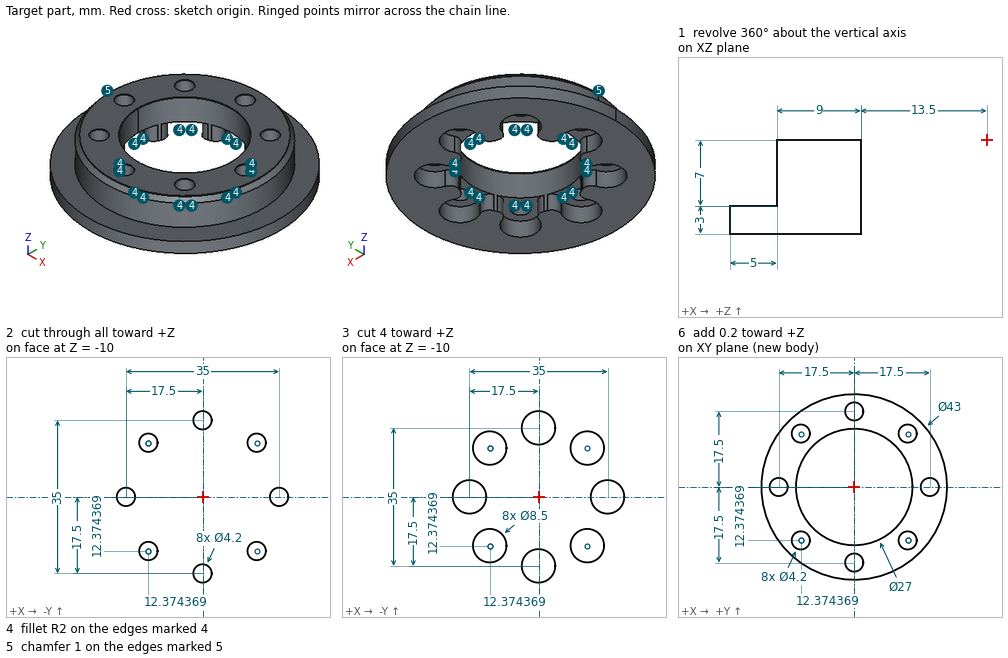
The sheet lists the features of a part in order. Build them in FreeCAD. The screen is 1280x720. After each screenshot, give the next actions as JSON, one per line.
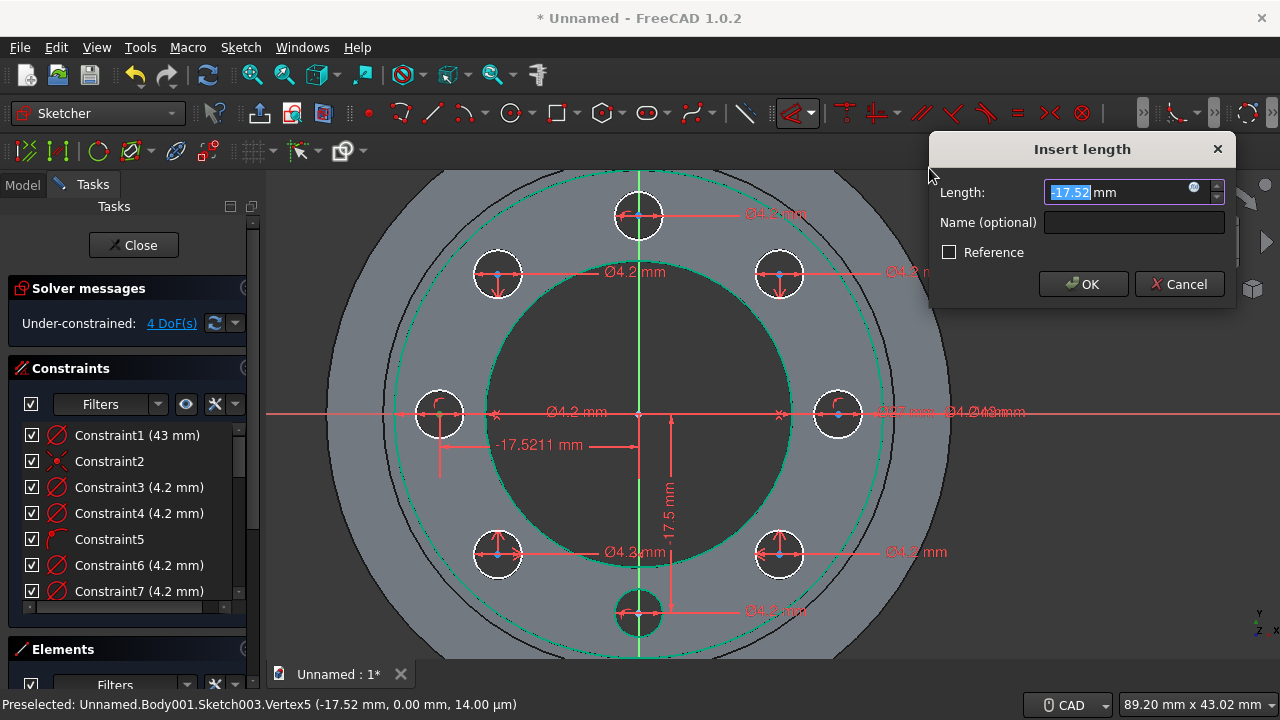
{"action": "type", "text": "-17.5"}
{"action": "key", "text": "Return"}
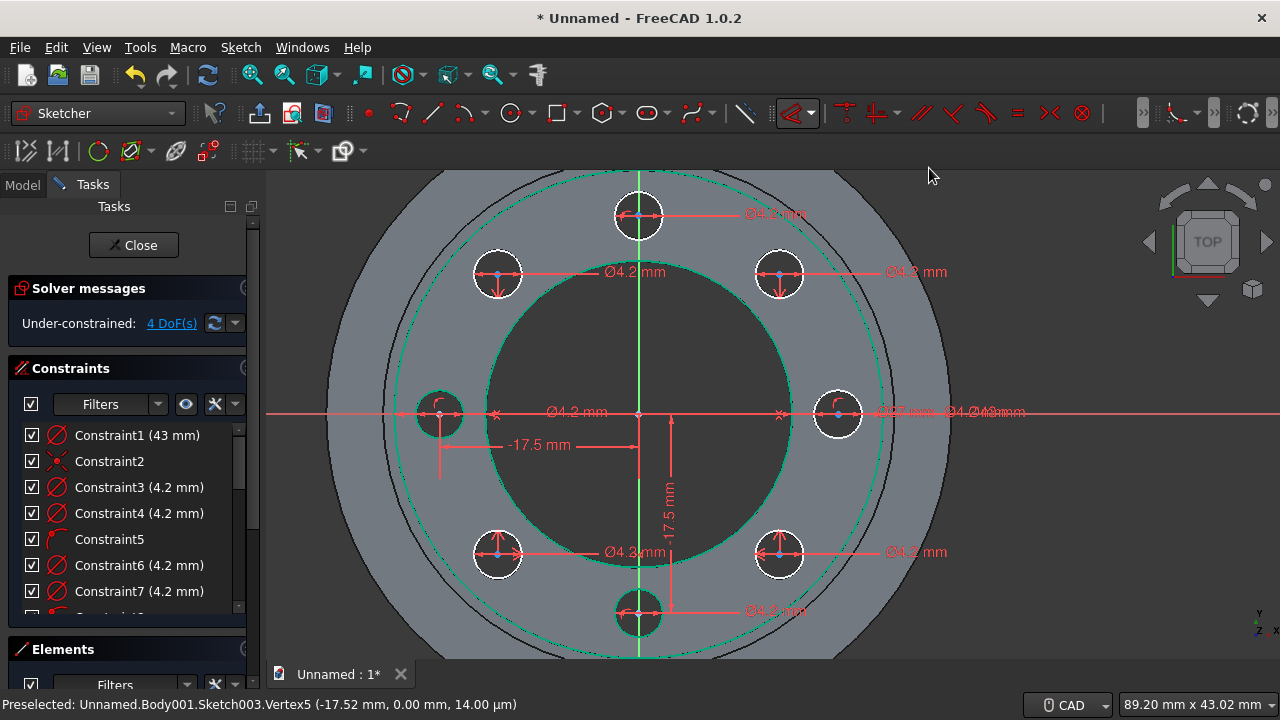
{"action": "left_click", "coordinate": [838, 414]}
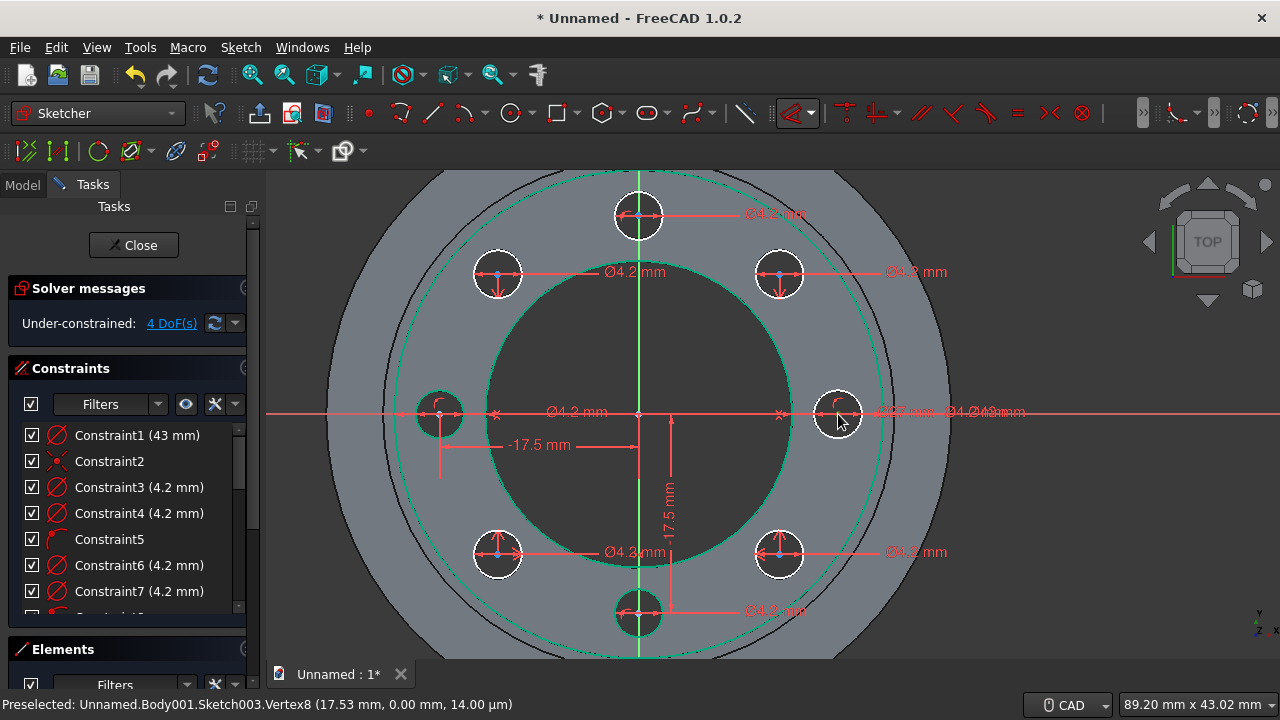
{"action": "key", "text": "l"}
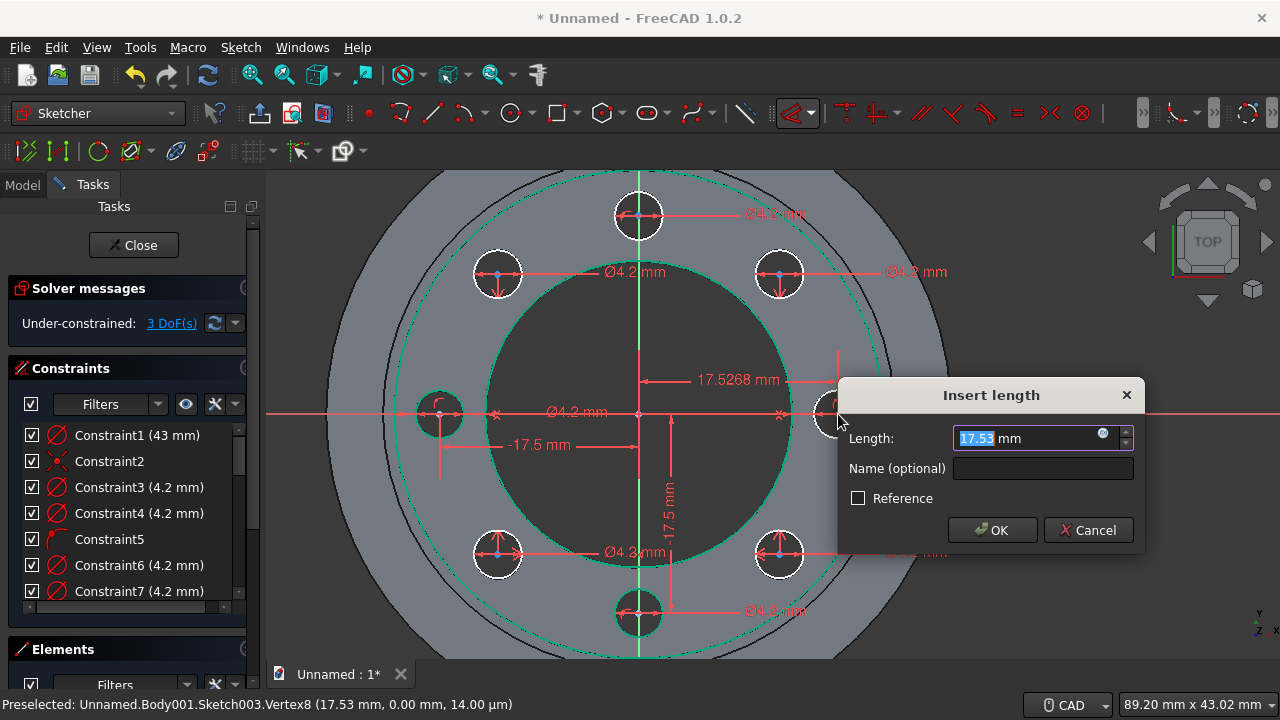
{"action": "type", "text": "17.5"}
{"action": "key", "text": "Return"}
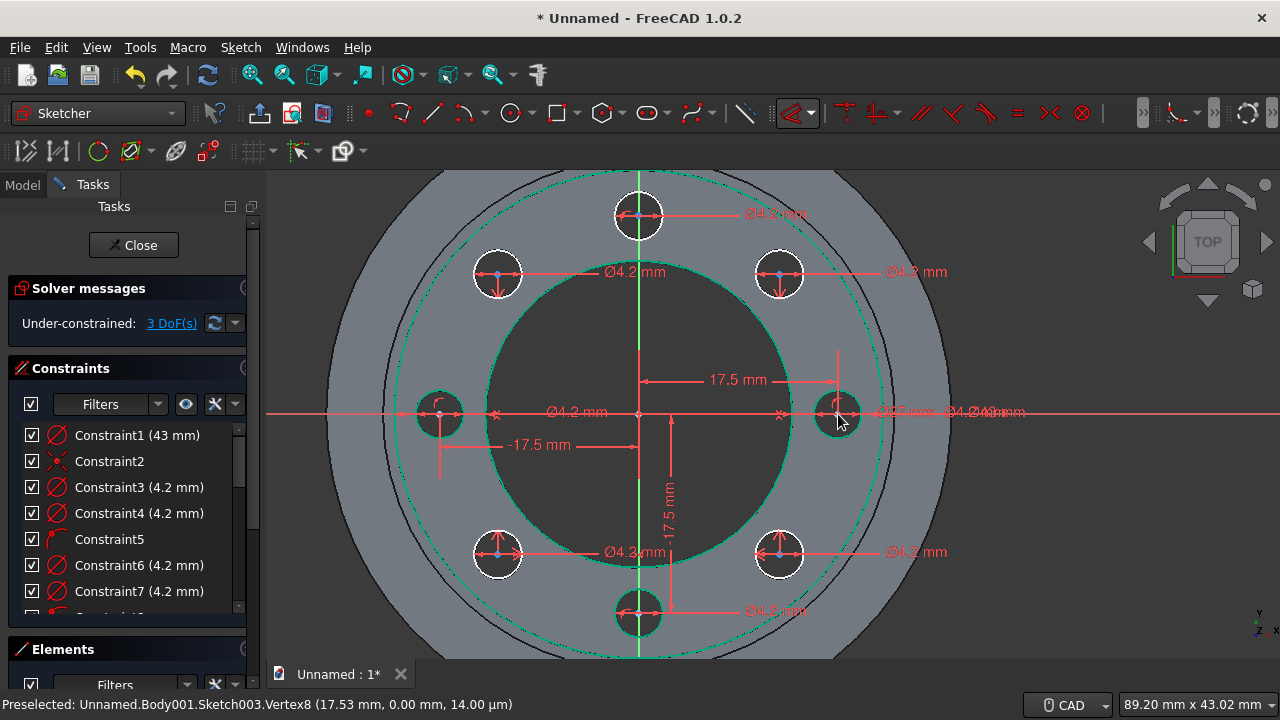
{"action": "left_click", "coordinate": [639, 216]}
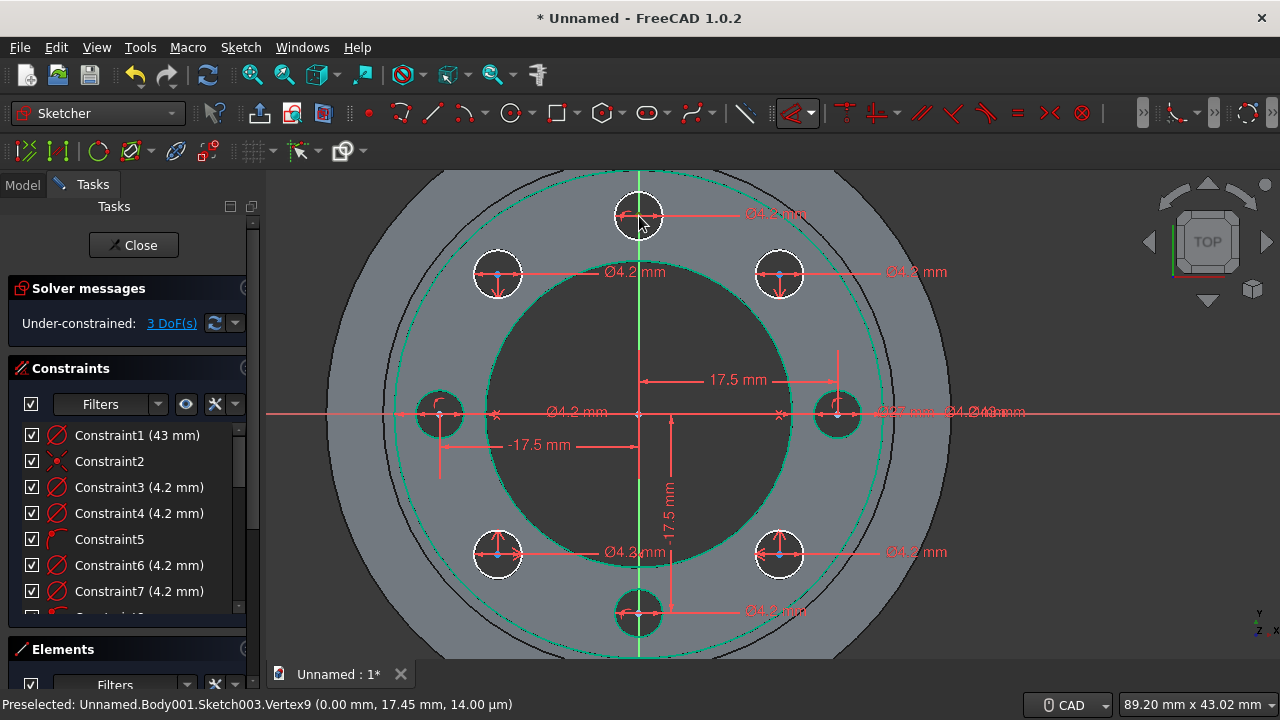
{"action": "key", "text": "i"}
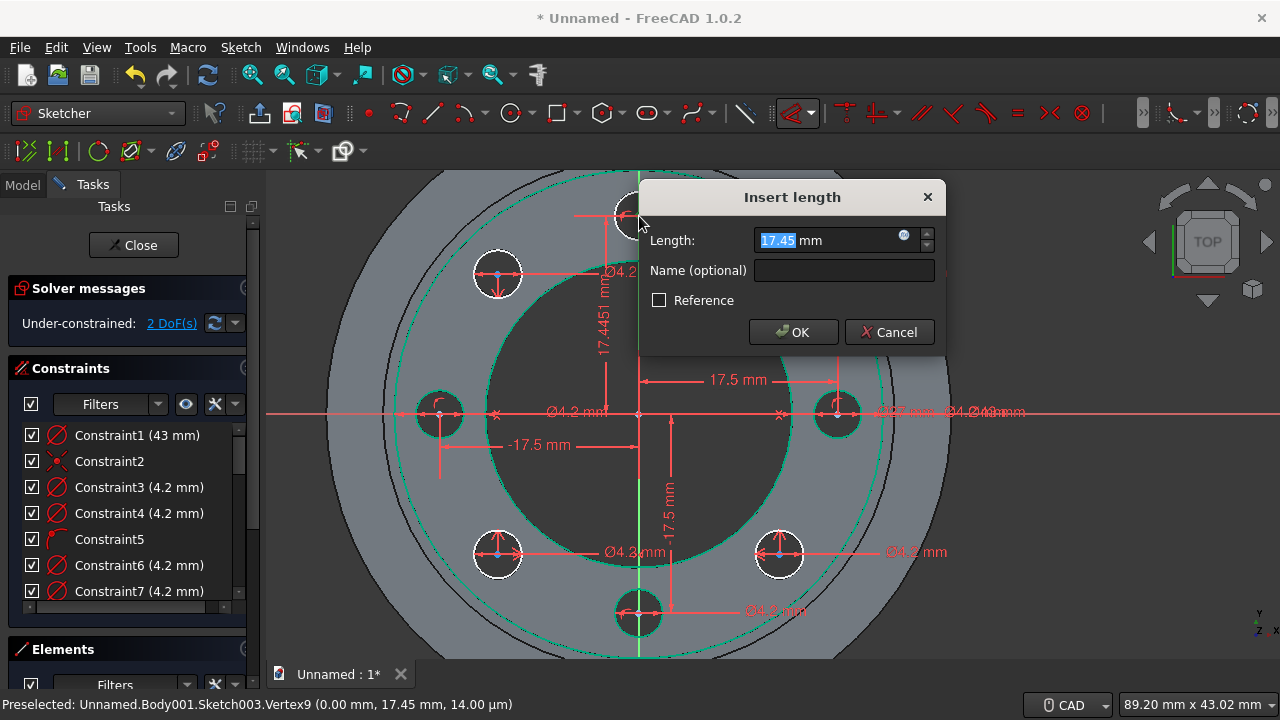
{"action": "type", "text": "17.5"}
{"action": "key", "text": "Return"}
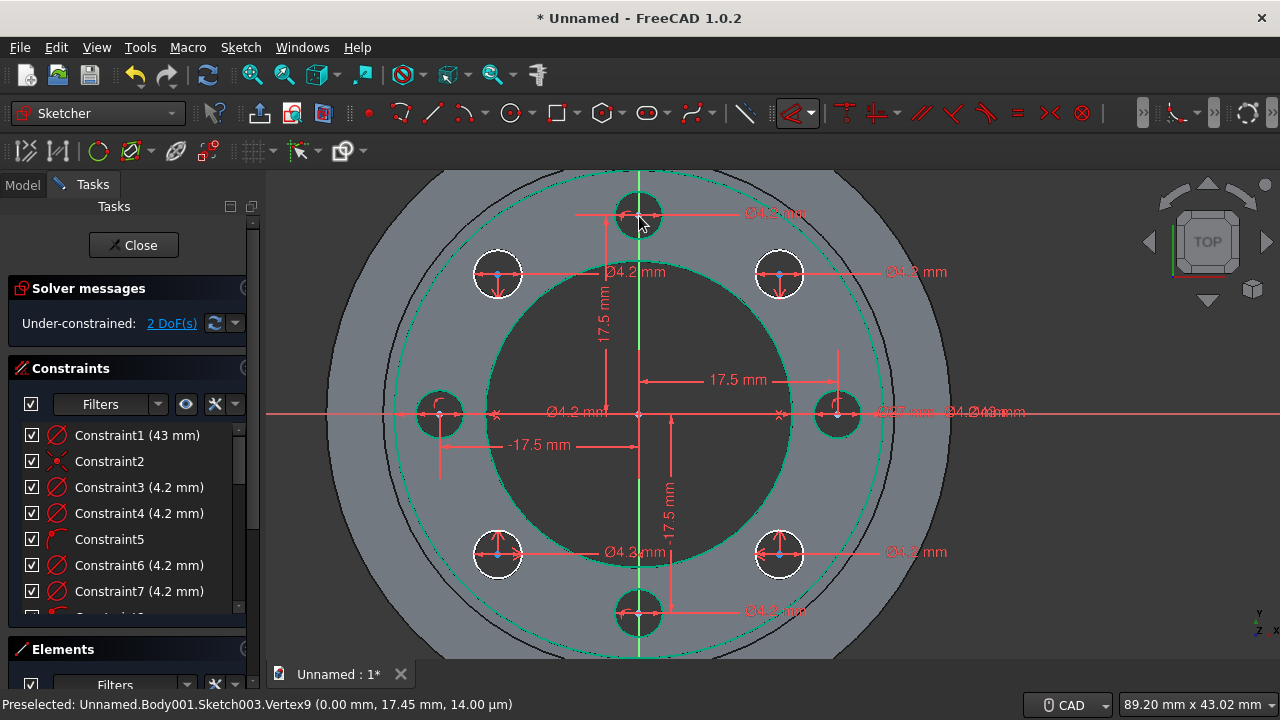
{"action": "left_click", "coordinate": [498, 554]}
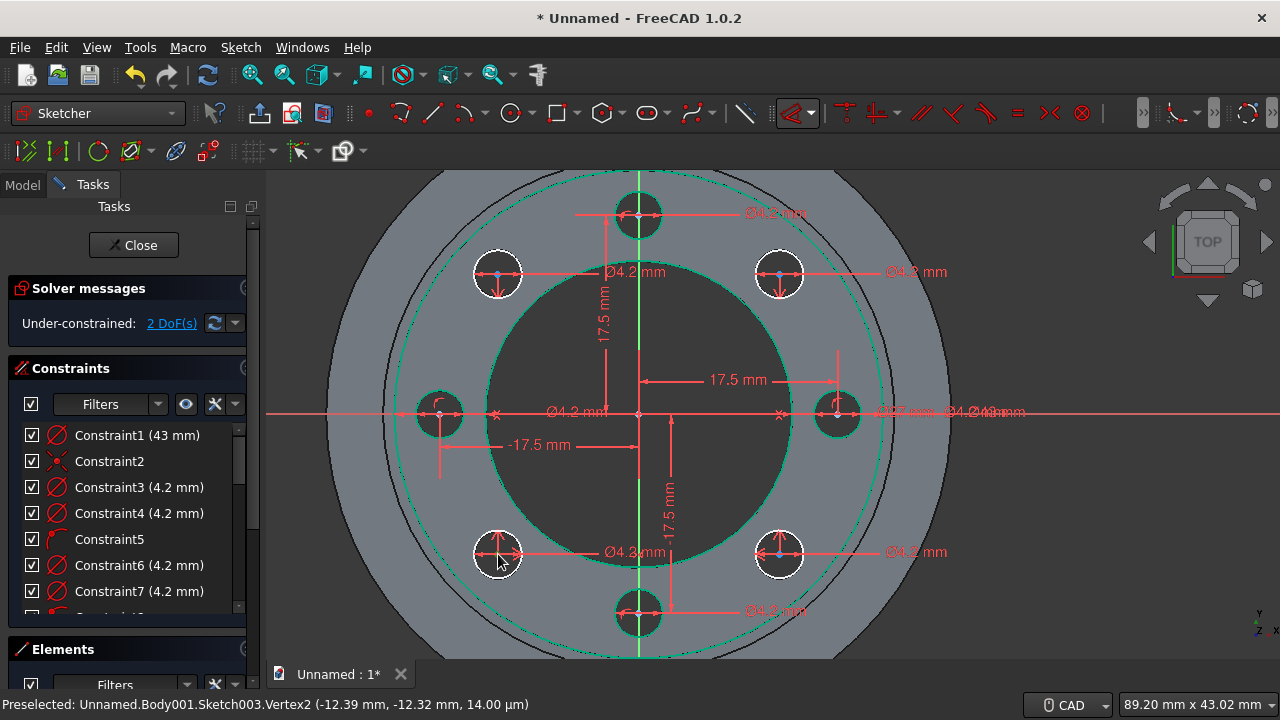
{"action": "key", "text": "l"}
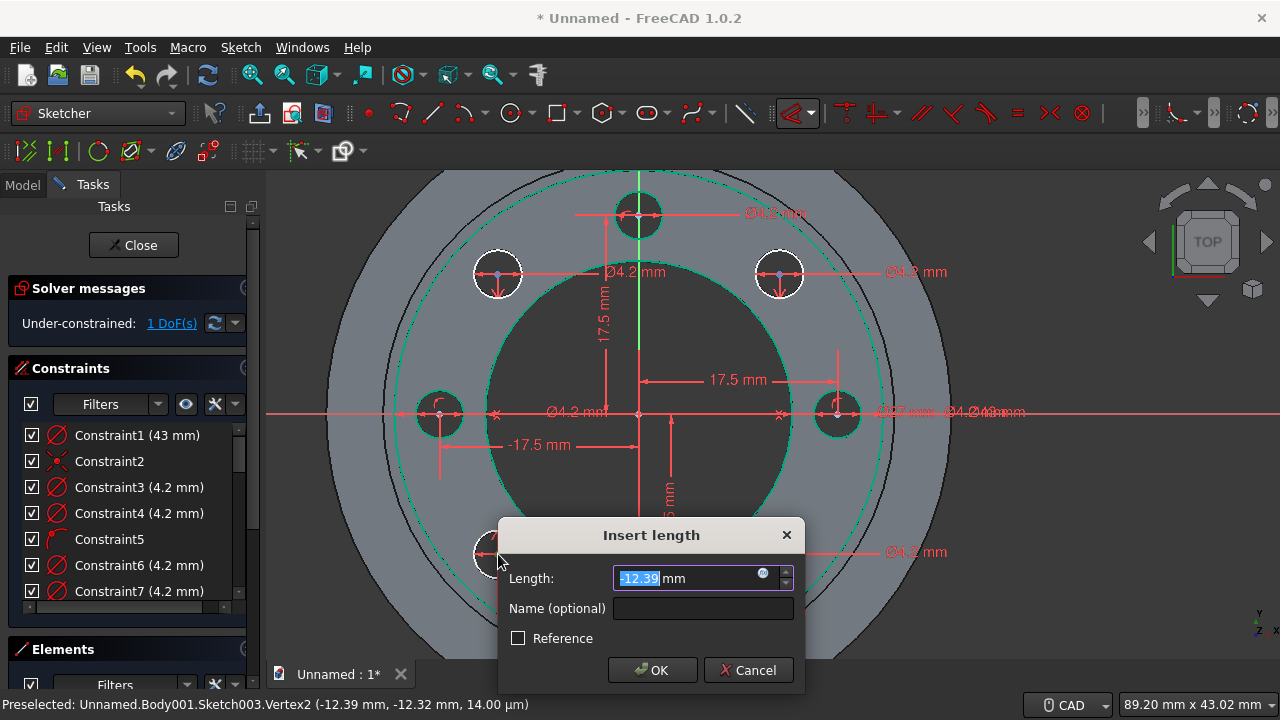
{"action": "type", "text": "-12.374369"}
{"action": "key", "text": "Return"}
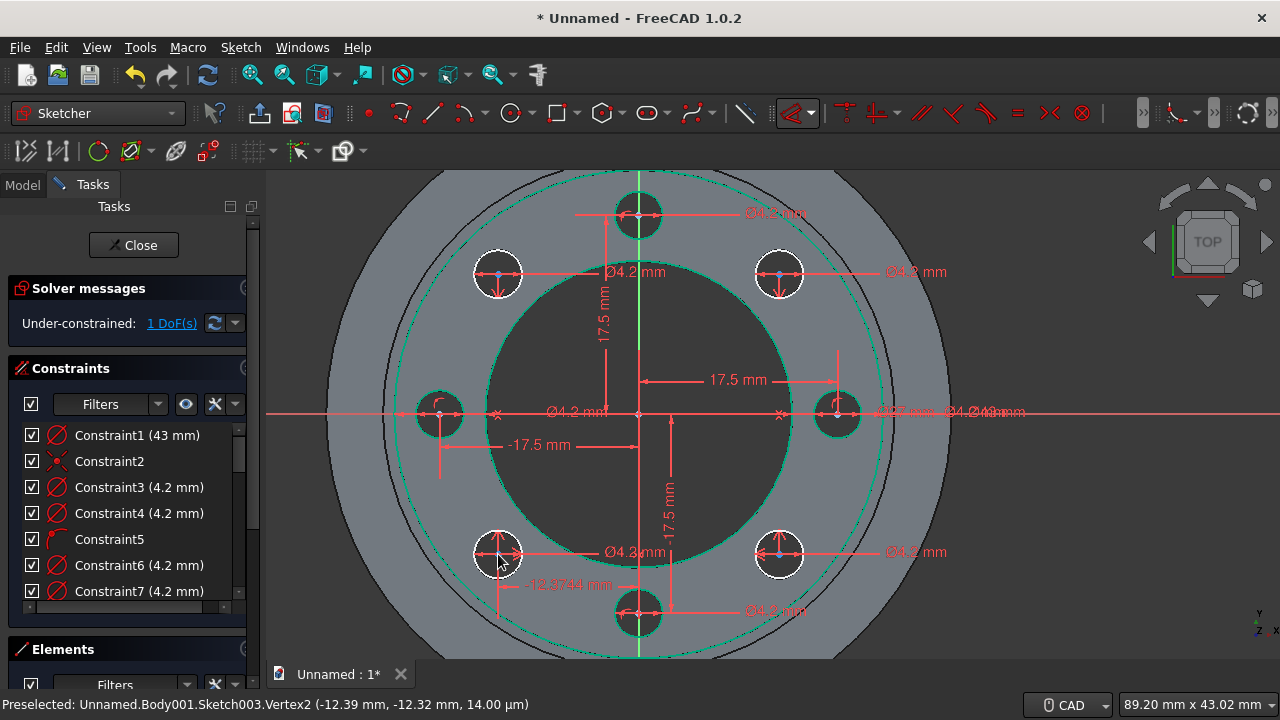
{"action": "left_click", "coordinate": [498, 554]}